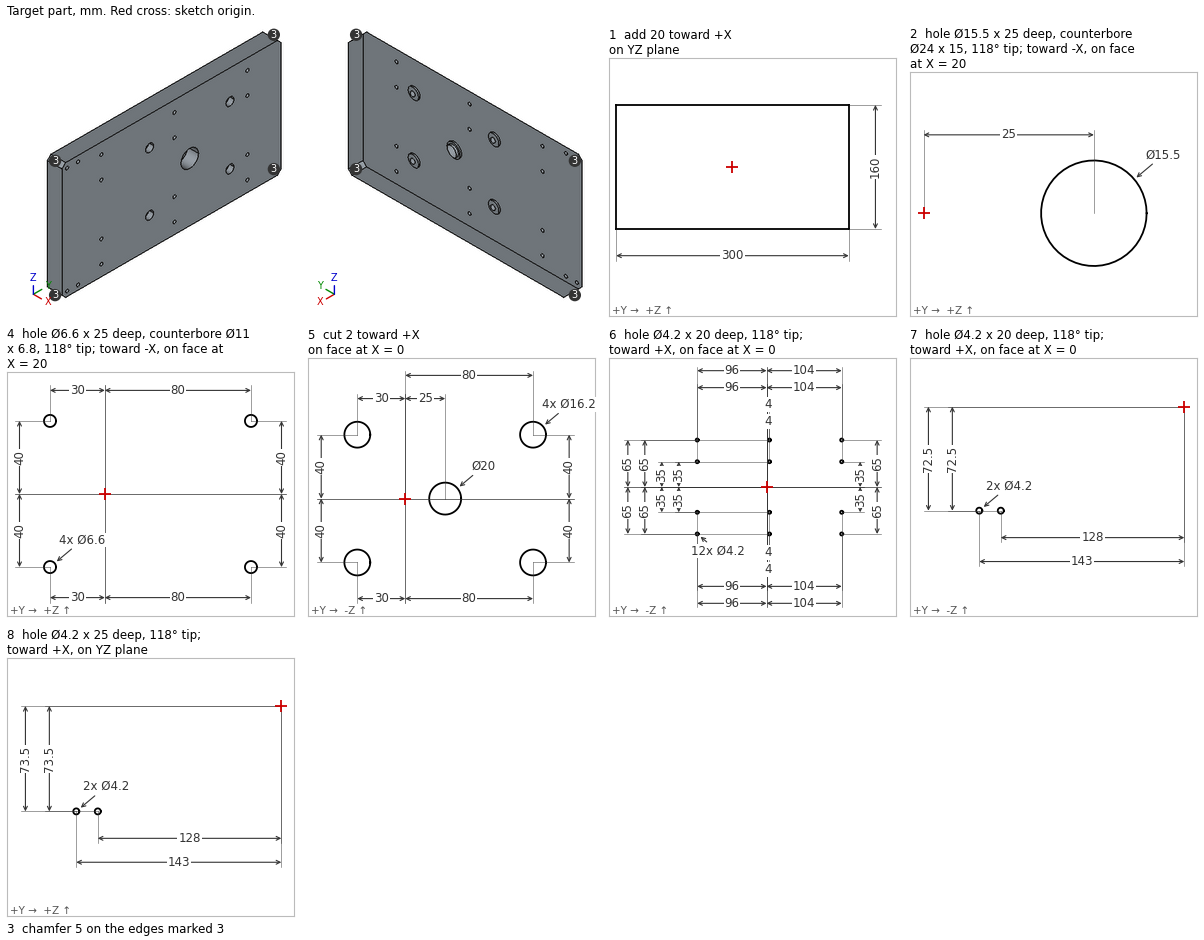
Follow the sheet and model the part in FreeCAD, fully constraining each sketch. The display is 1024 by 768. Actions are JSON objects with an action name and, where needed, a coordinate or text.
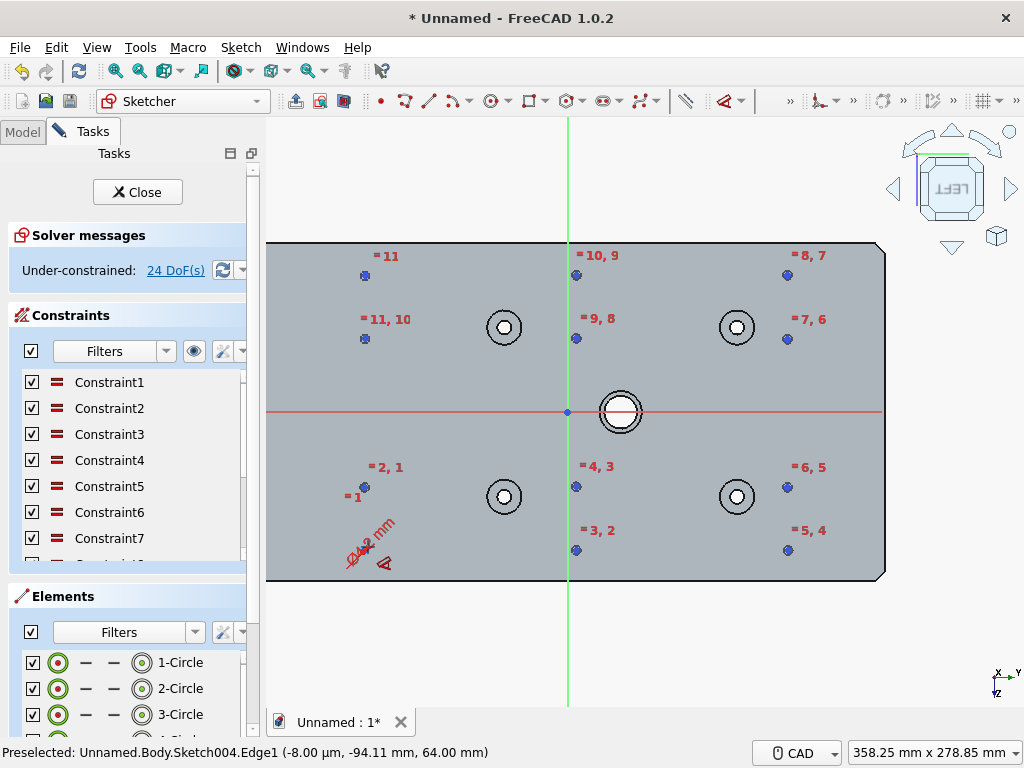
{"action": "scroll", "coordinate": [576, 550], "scroll_direction": "up", "scroll_amount": 8}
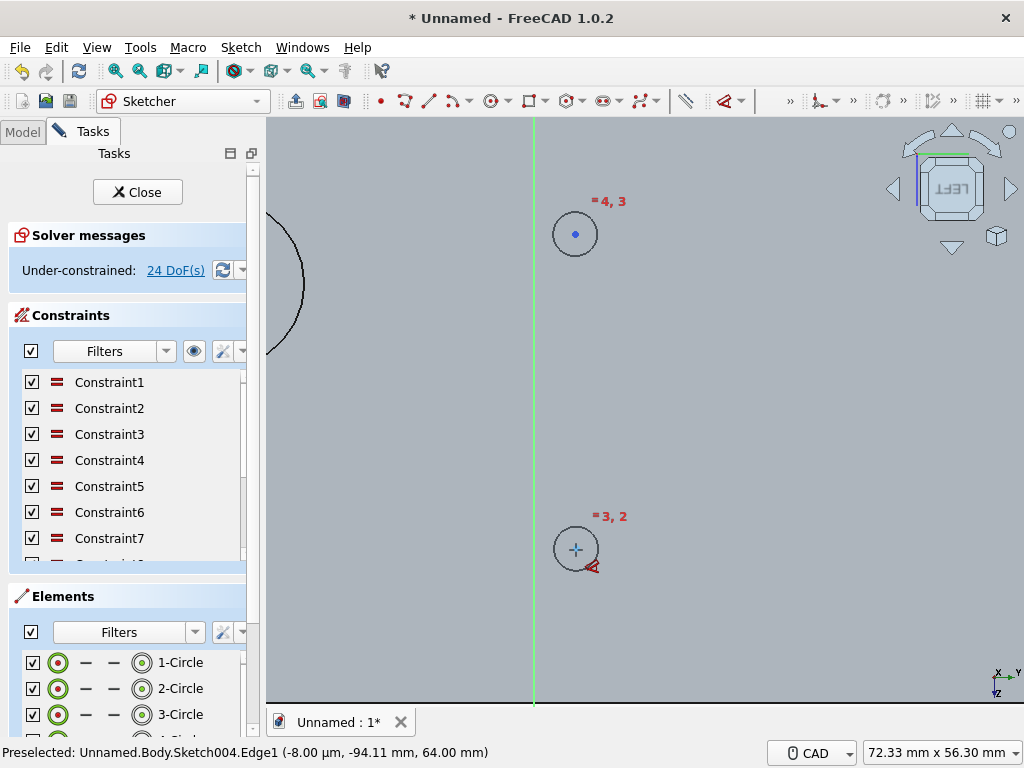
{"action": "left_click", "coordinate": [576, 549]}
{"action": "left_click", "coordinate": [555, 583]}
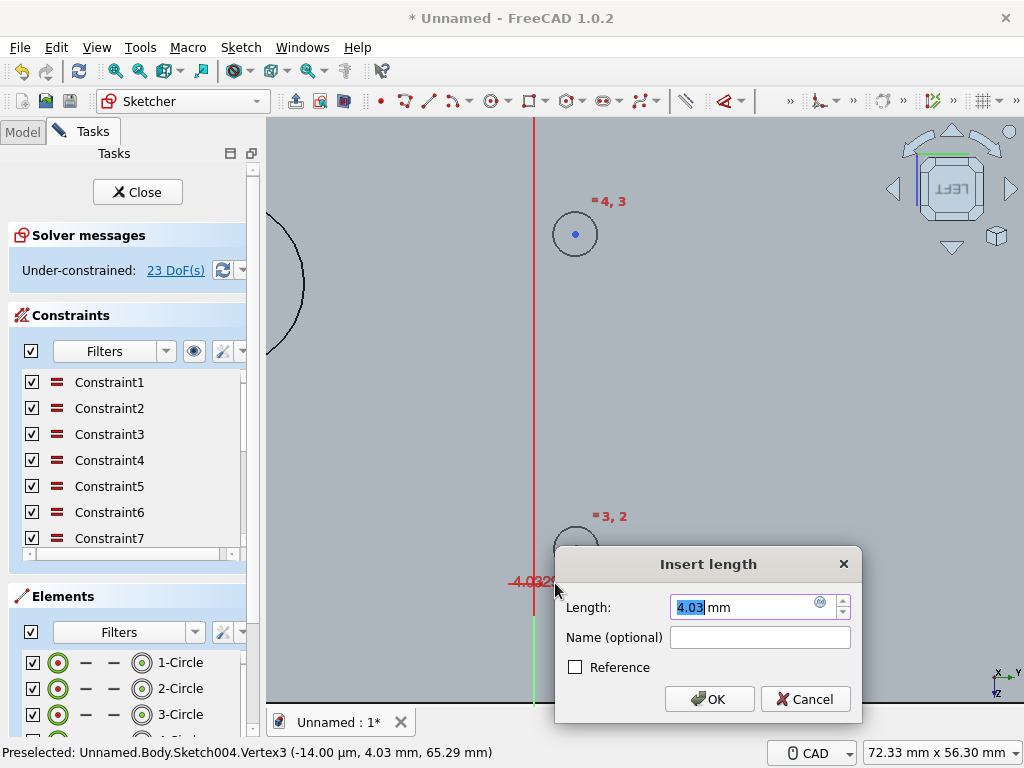
{"action": "type", "text": "4"}
{"action": "key", "text": "Return"}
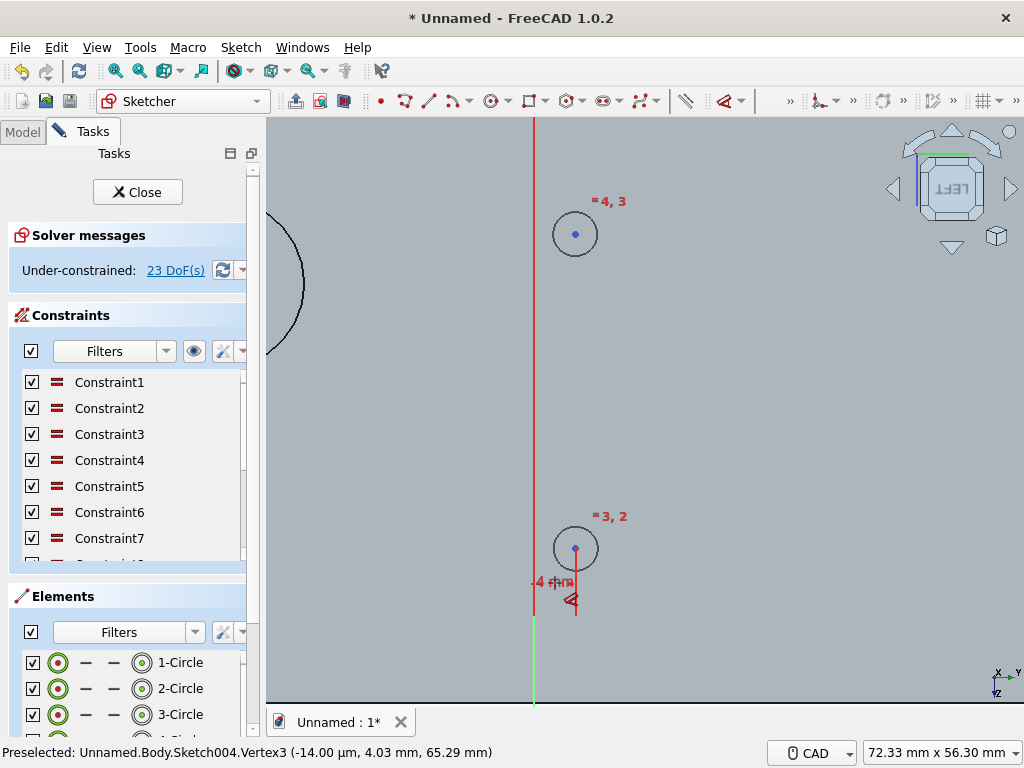
{"action": "left_click", "coordinate": [575, 234]}
{"action": "left_click", "coordinate": [555, 268]}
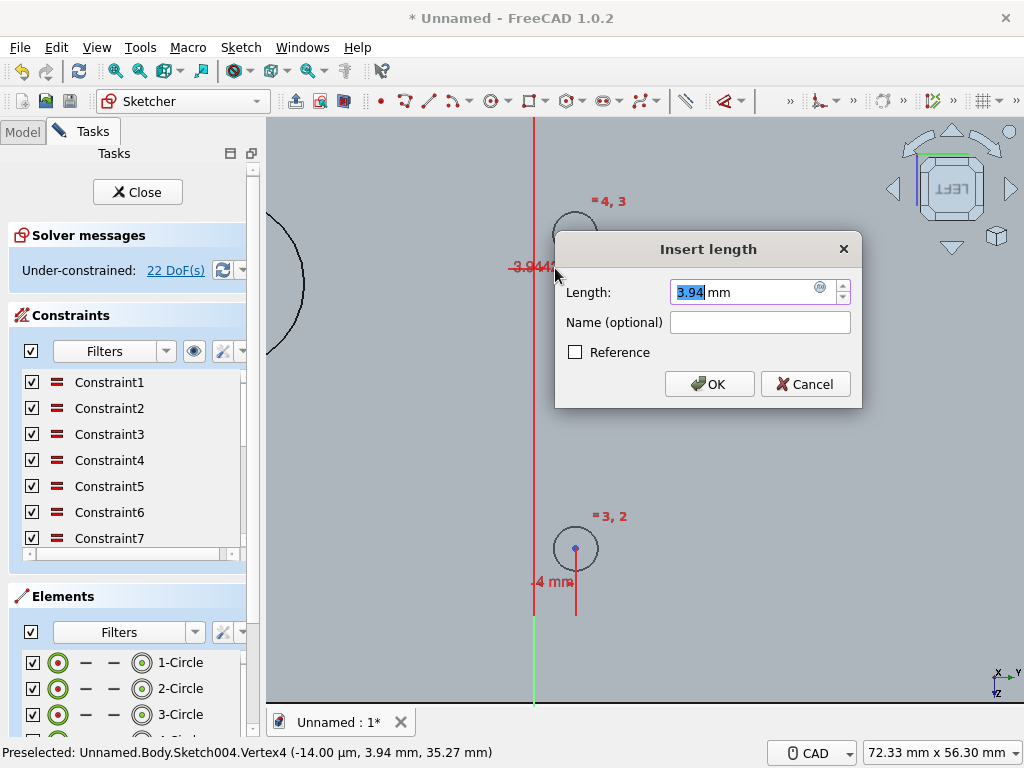
{"action": "type", "text": "4"}
{"action": "key", "text": "Return"}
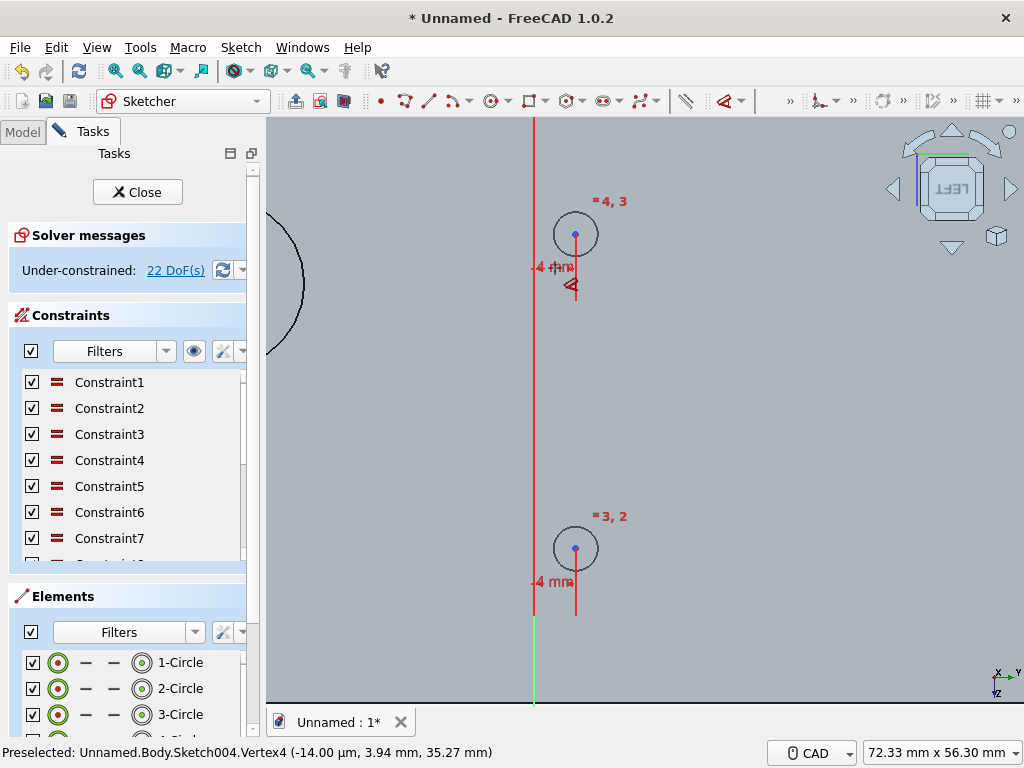
{"action": "scroll", "coordinate": [577, 550], "scroll_direction": "down", "scroll_amount": 8}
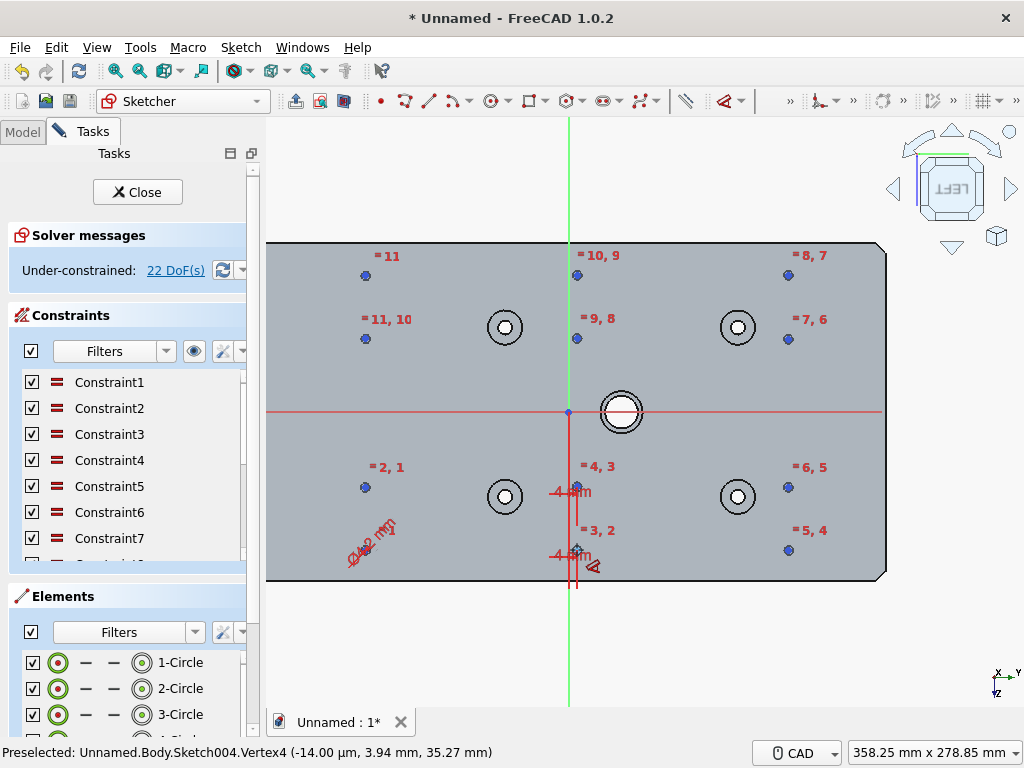
{"action": "scroll", "coordinate": [577, 338], "scroll_direction": "up", "scroll_amount": 8}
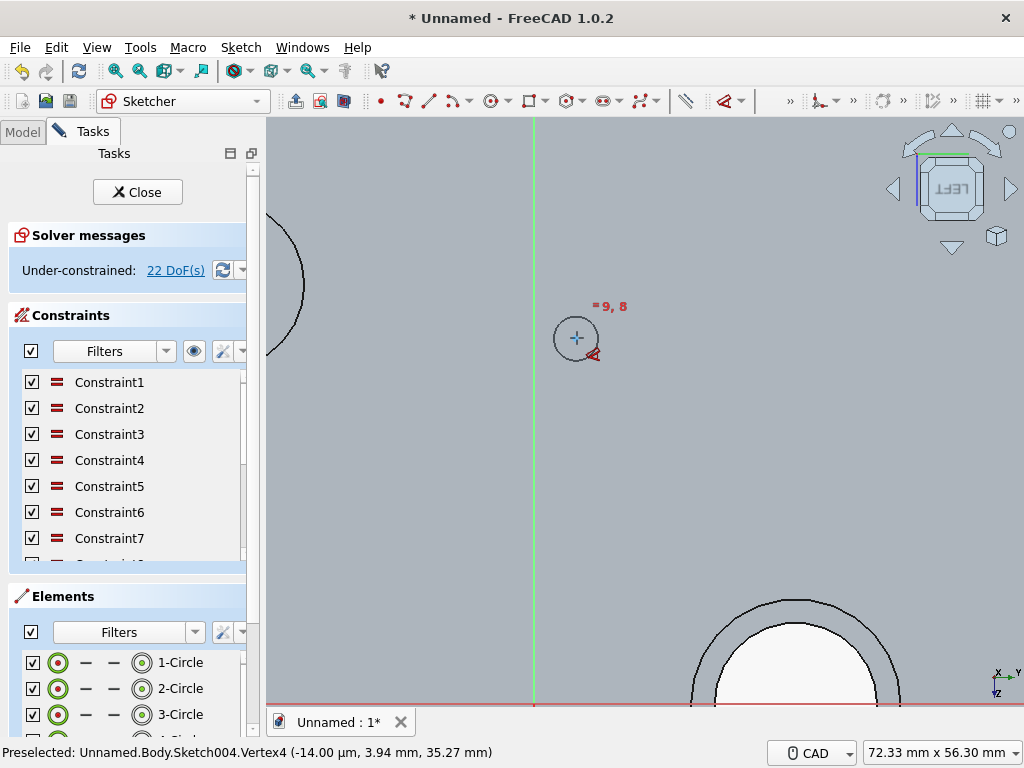
{"action": "left_click", "coordinate": [576, 339]}
{"action": "left_click", "coordinate": [555, 305]}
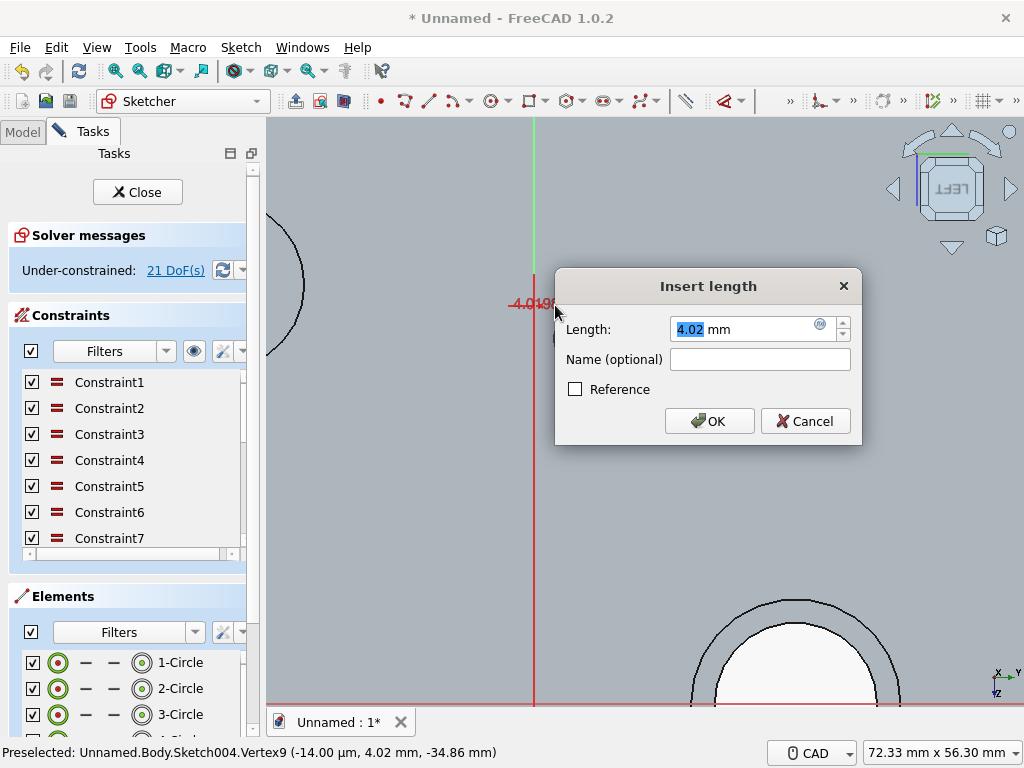
{"action": "type", "text": "4"}
{"action": "key", "text": "Return"}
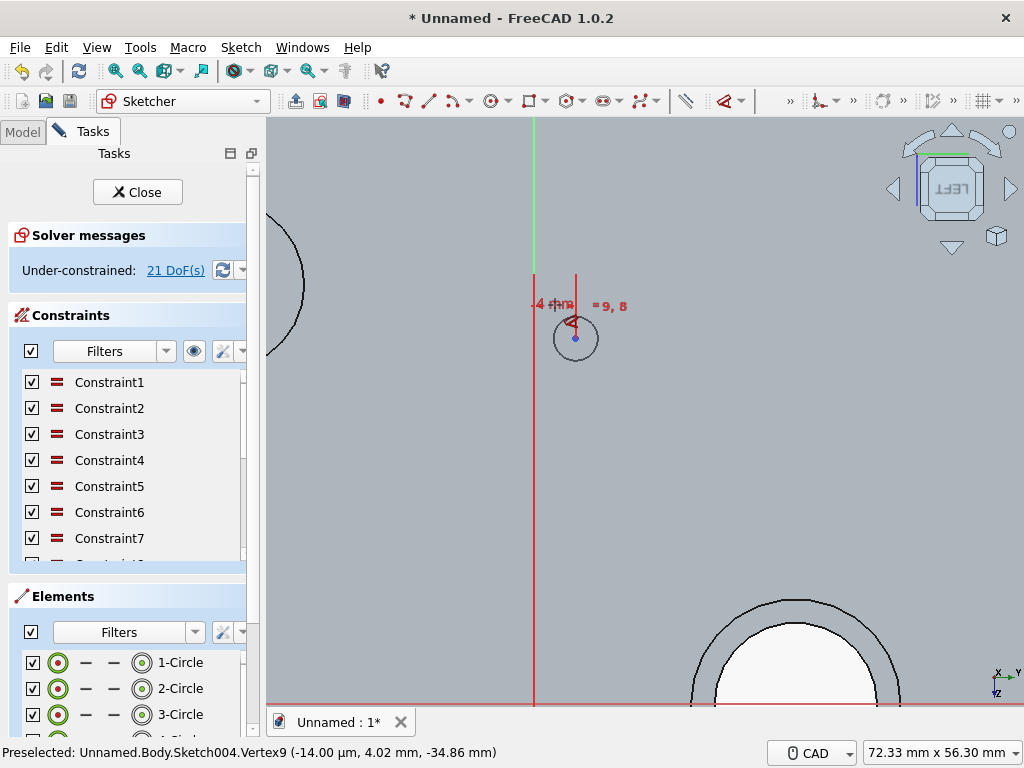
{"action": "scroll", "coordinate": [577, 338], "scroll_direction": "down", "scroll_amount": 8}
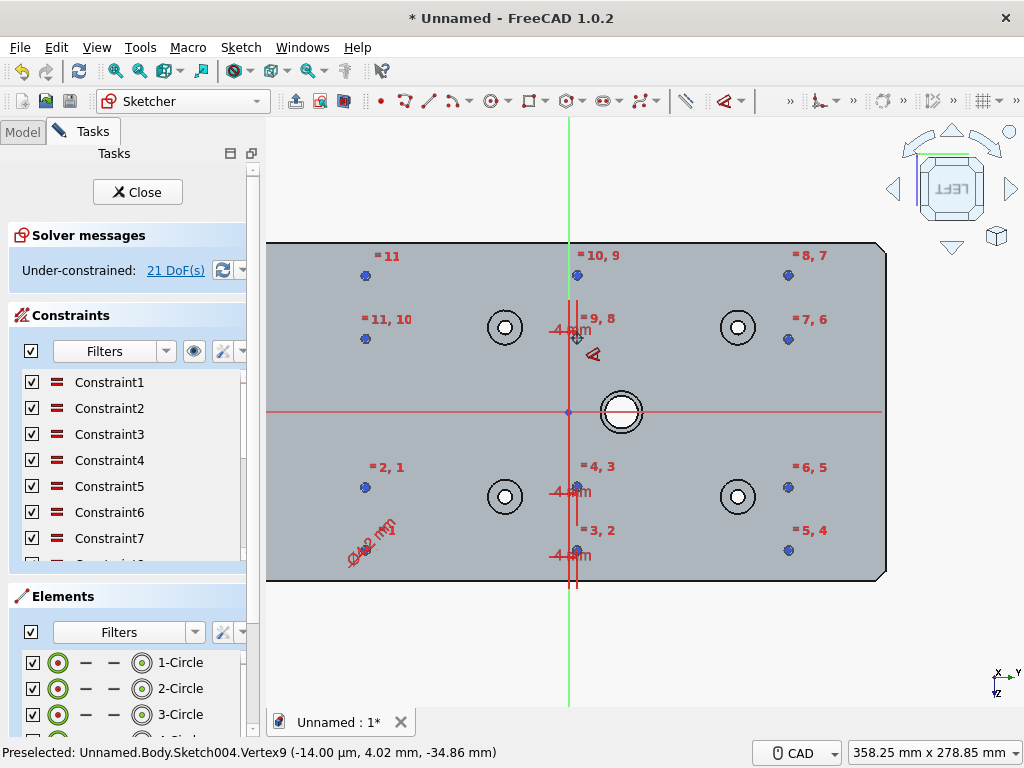
{"action": "scroll", "coordinate": [577, 275], "scroll_direction": "up", "scroll_amount": 8}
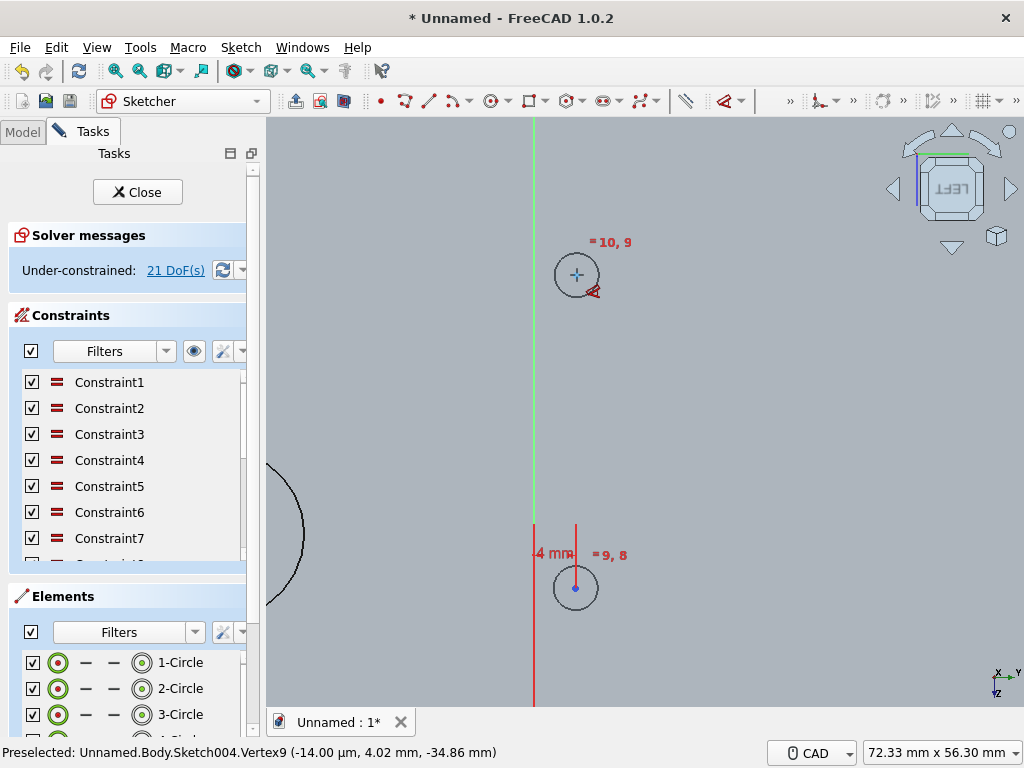
{"action": "left_click", "coordinate": [577, 275]}
{"action": "left_click", "coordinate": [555, 241]}